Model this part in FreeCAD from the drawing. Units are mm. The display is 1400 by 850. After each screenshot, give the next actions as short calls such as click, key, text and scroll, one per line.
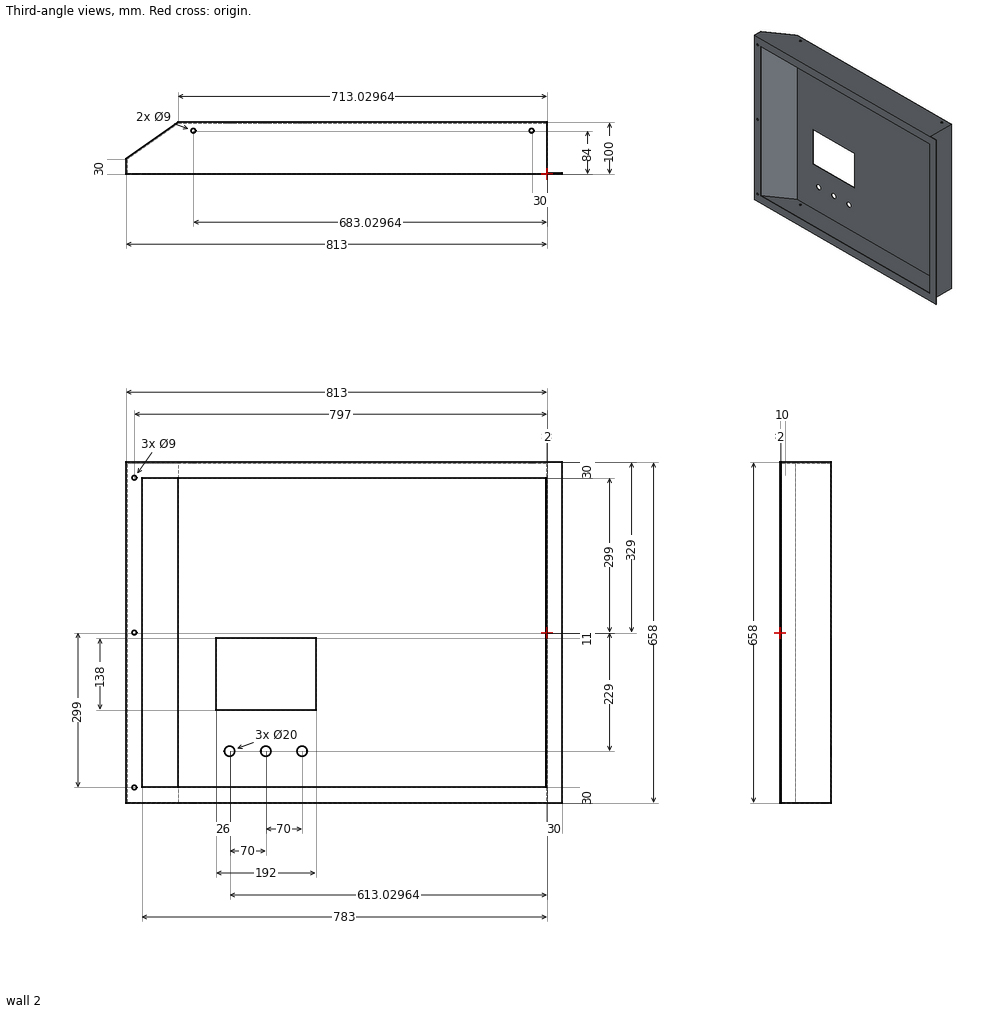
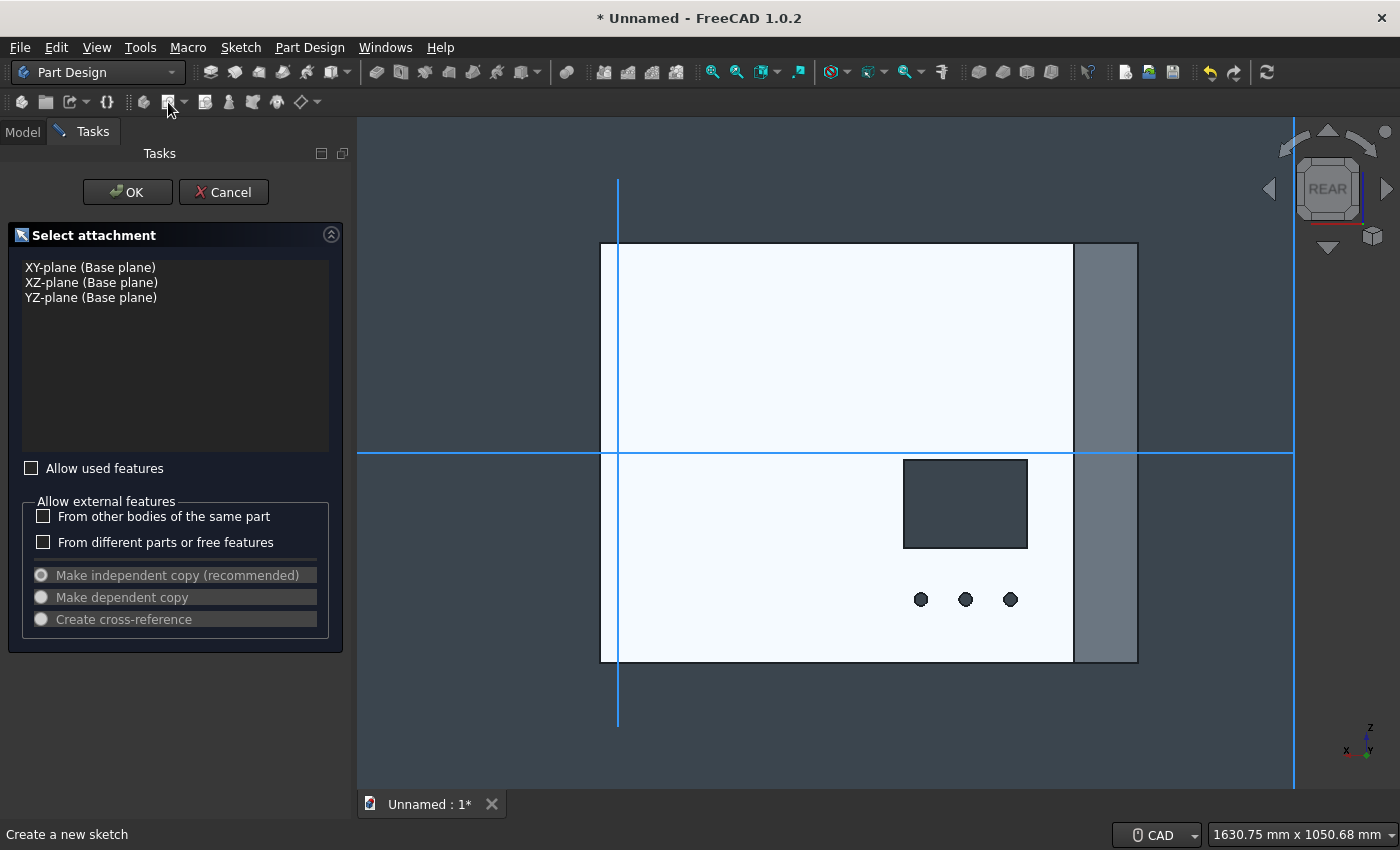
click(82, 282)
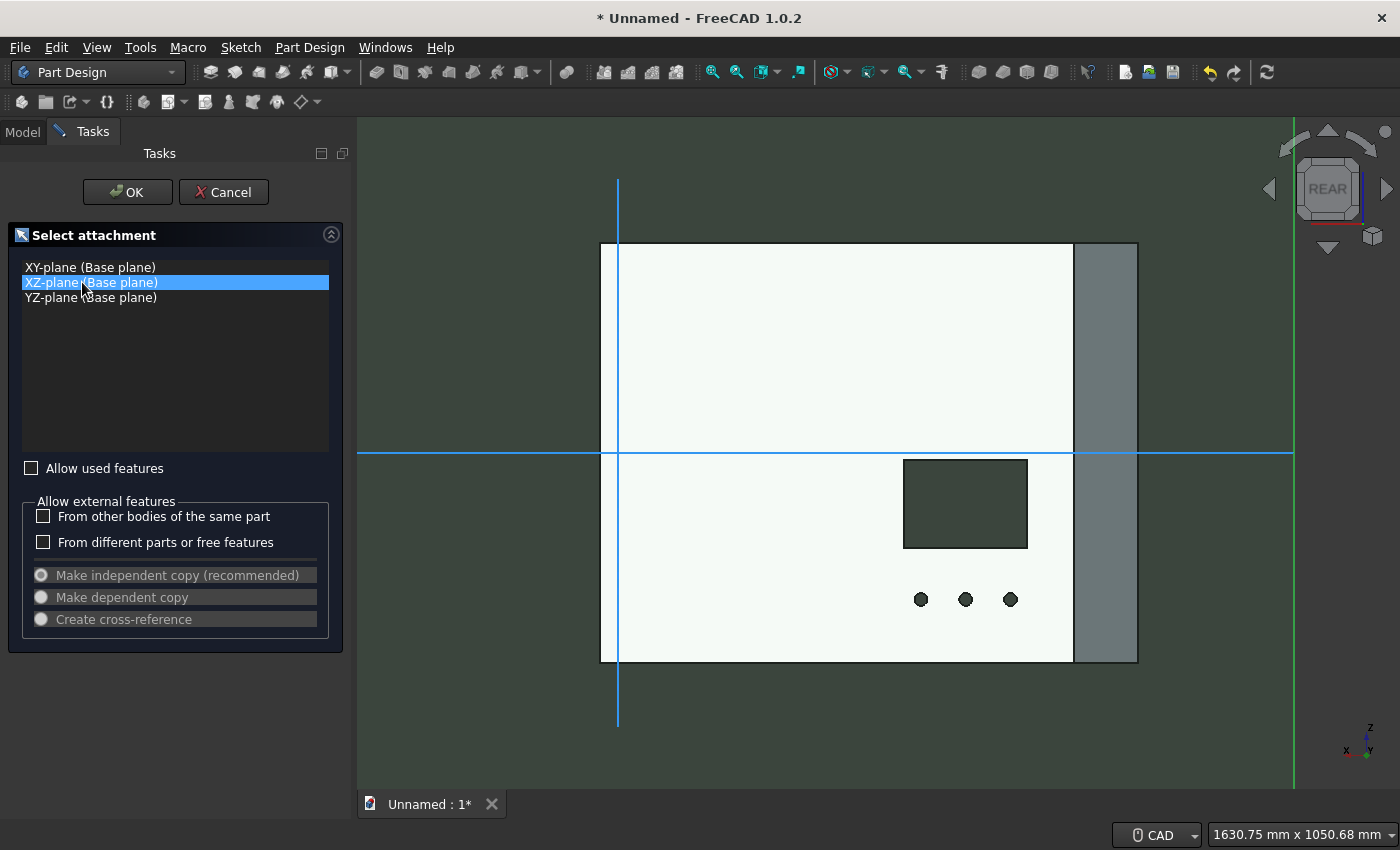
click(128, 192)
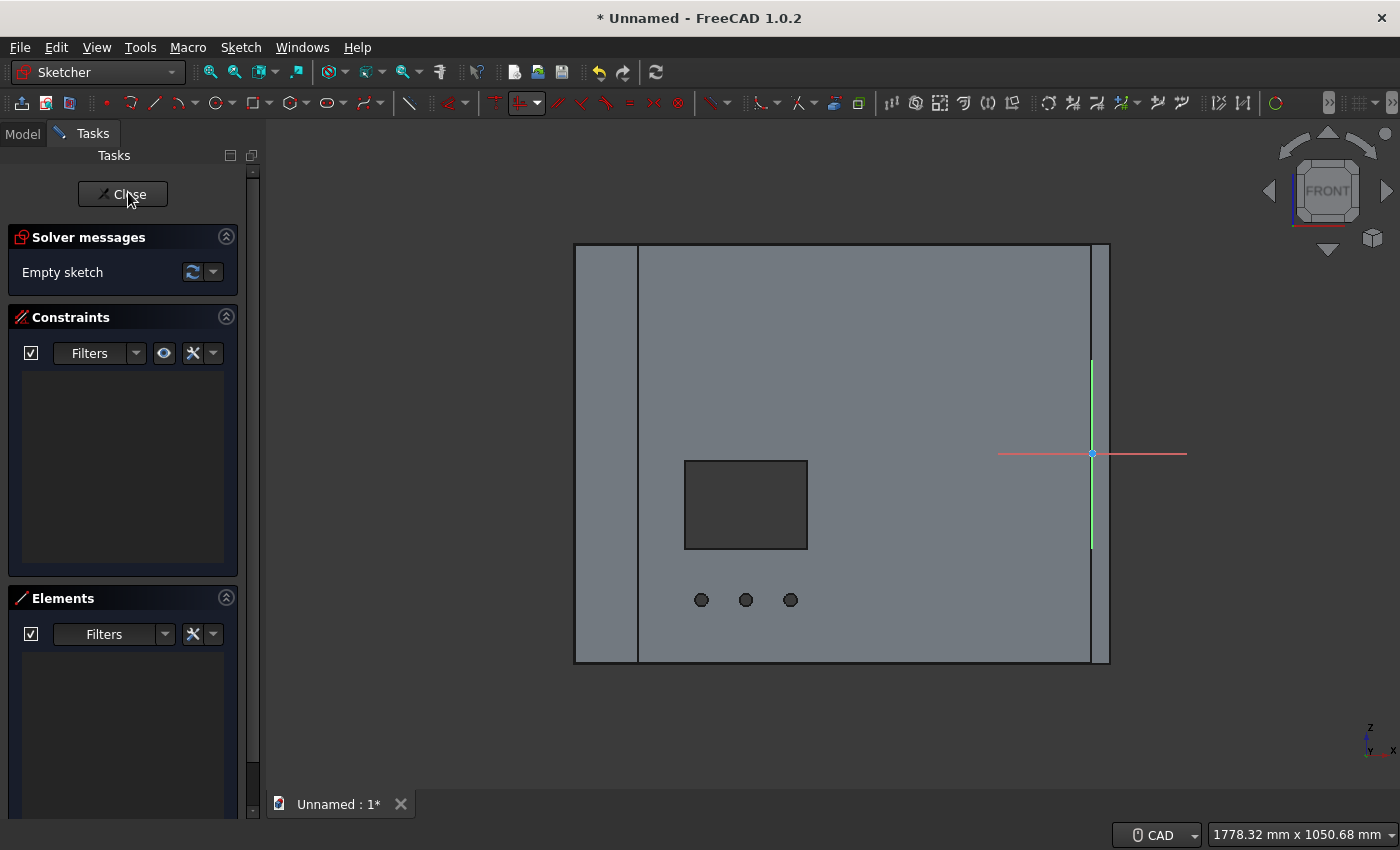
click(132, 104)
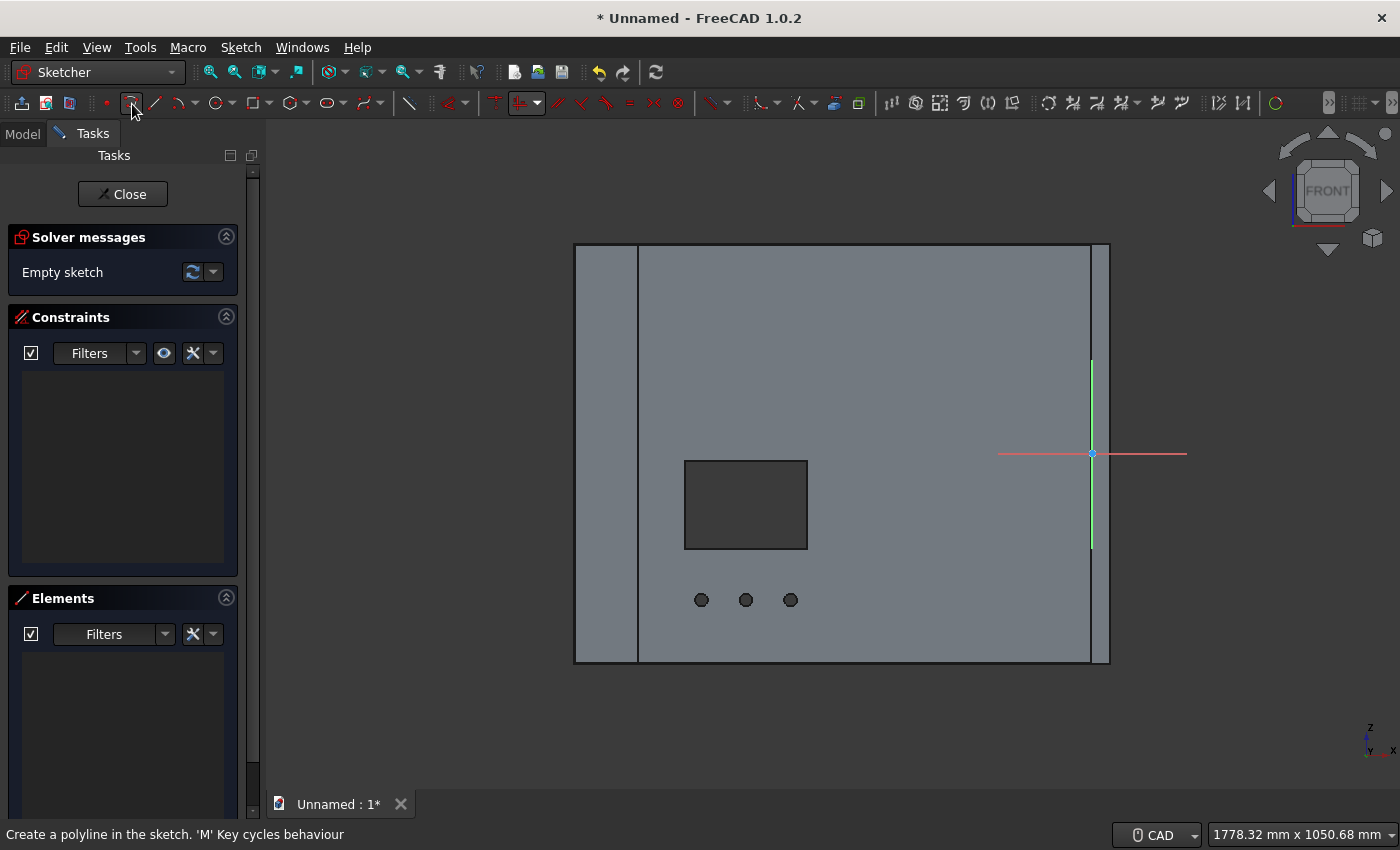
click(1092, 263)
click(1083, 244)
click(574, 244)
click(574, 664)
click(1092, 664)
click(1083, 645)
click(593, 645)
click(593, 263)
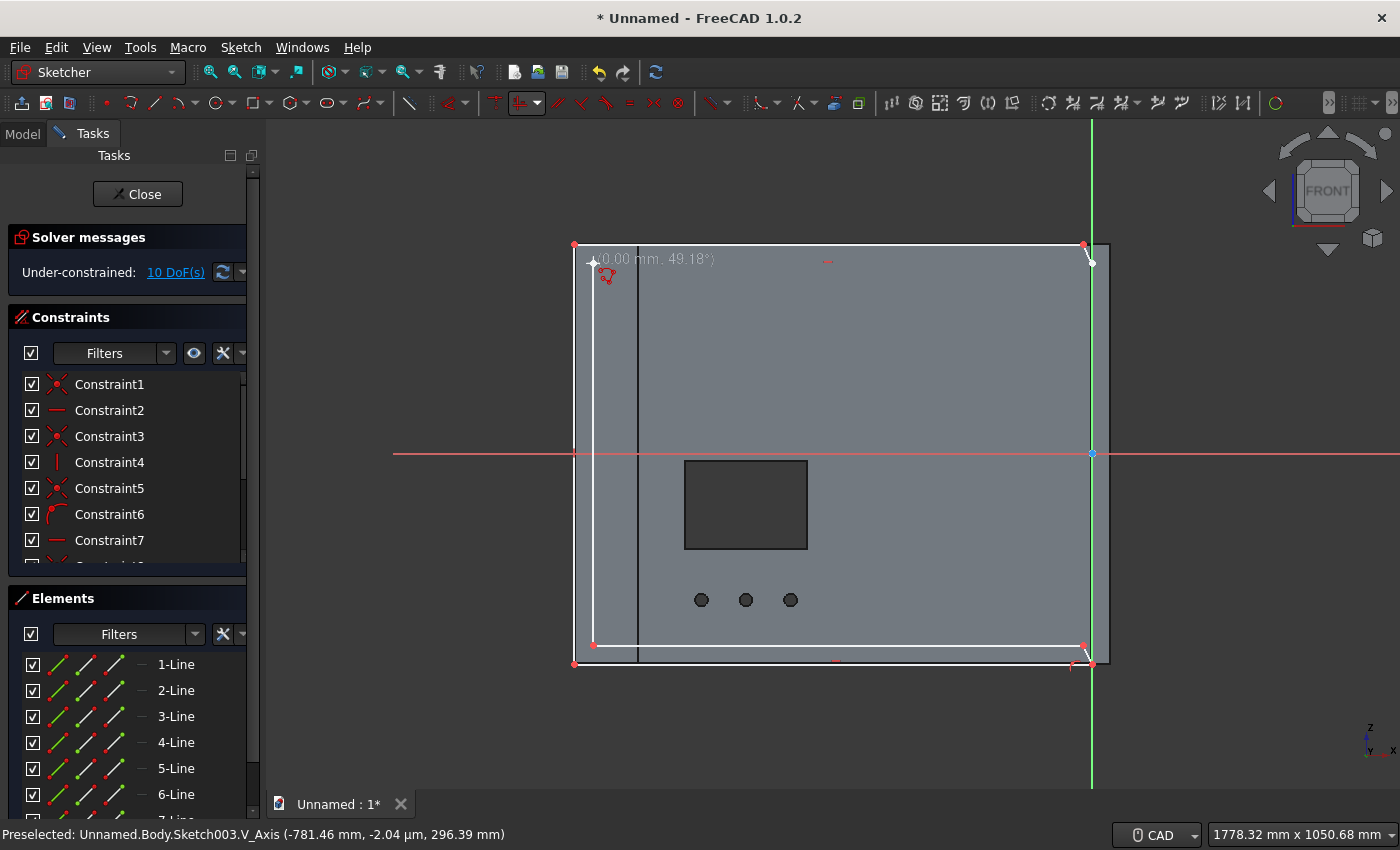
scroll(1092, 263, up, 3)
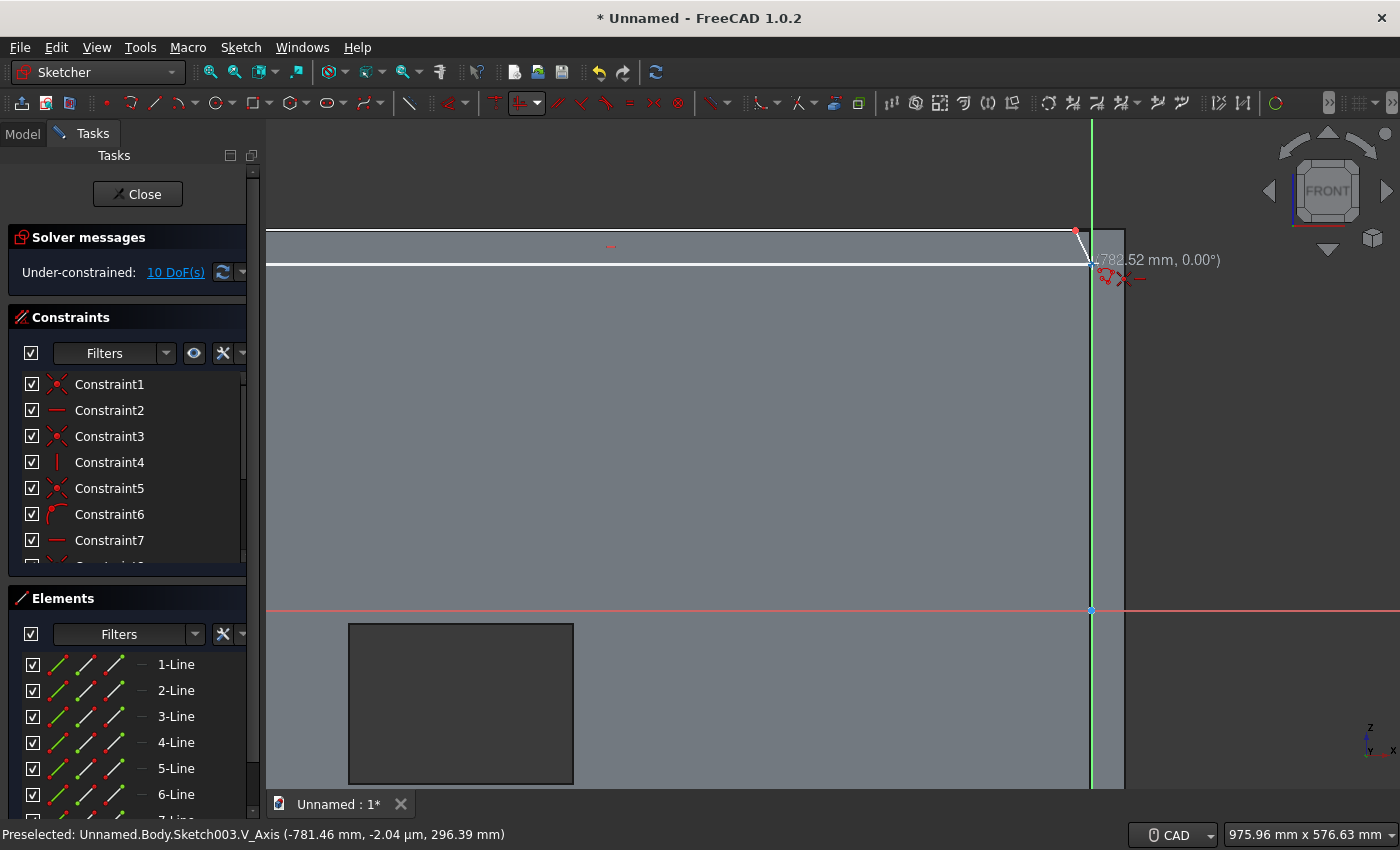
click(1091, 265)
key(Escape)
key(Escape)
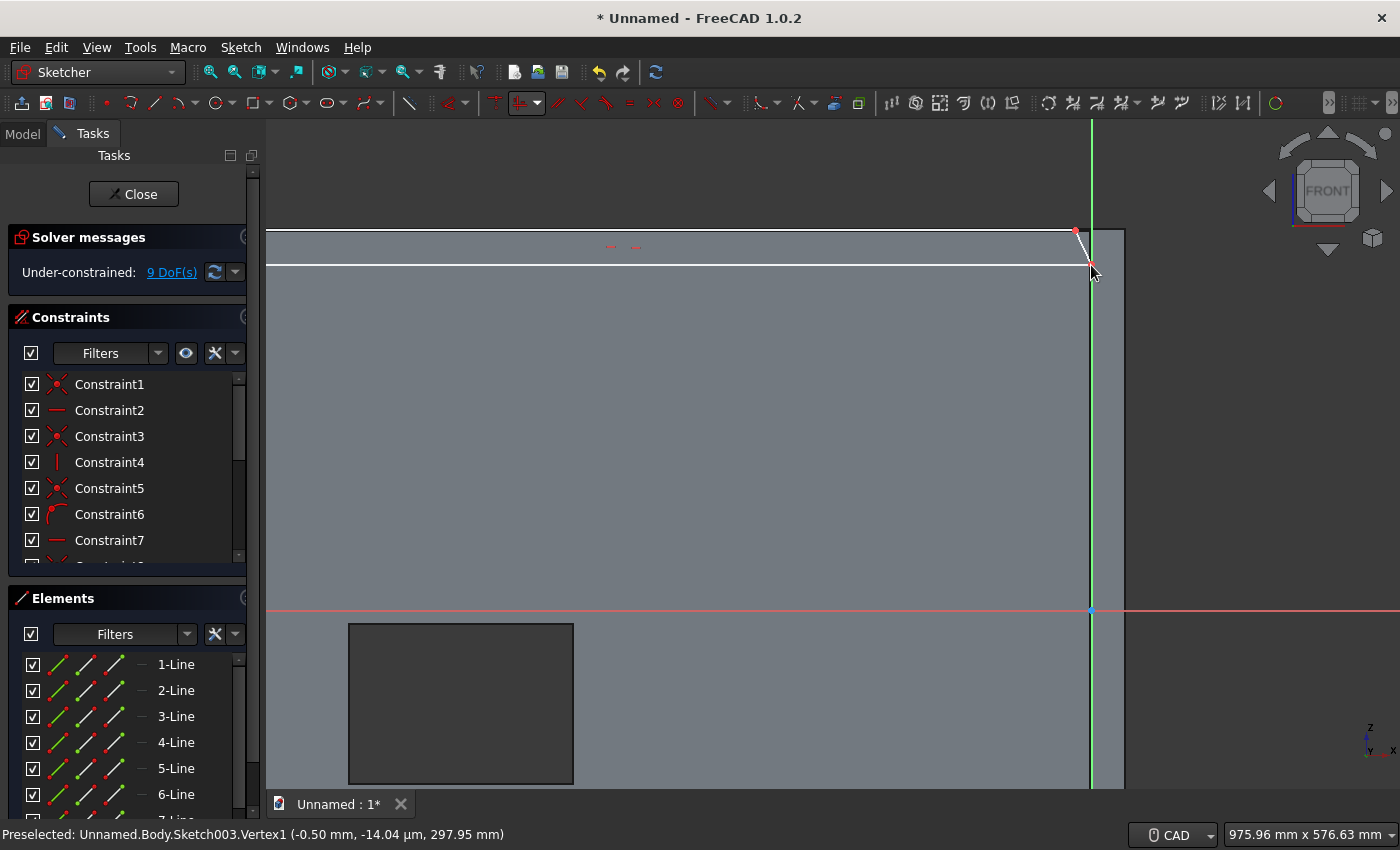
click(1080, 240)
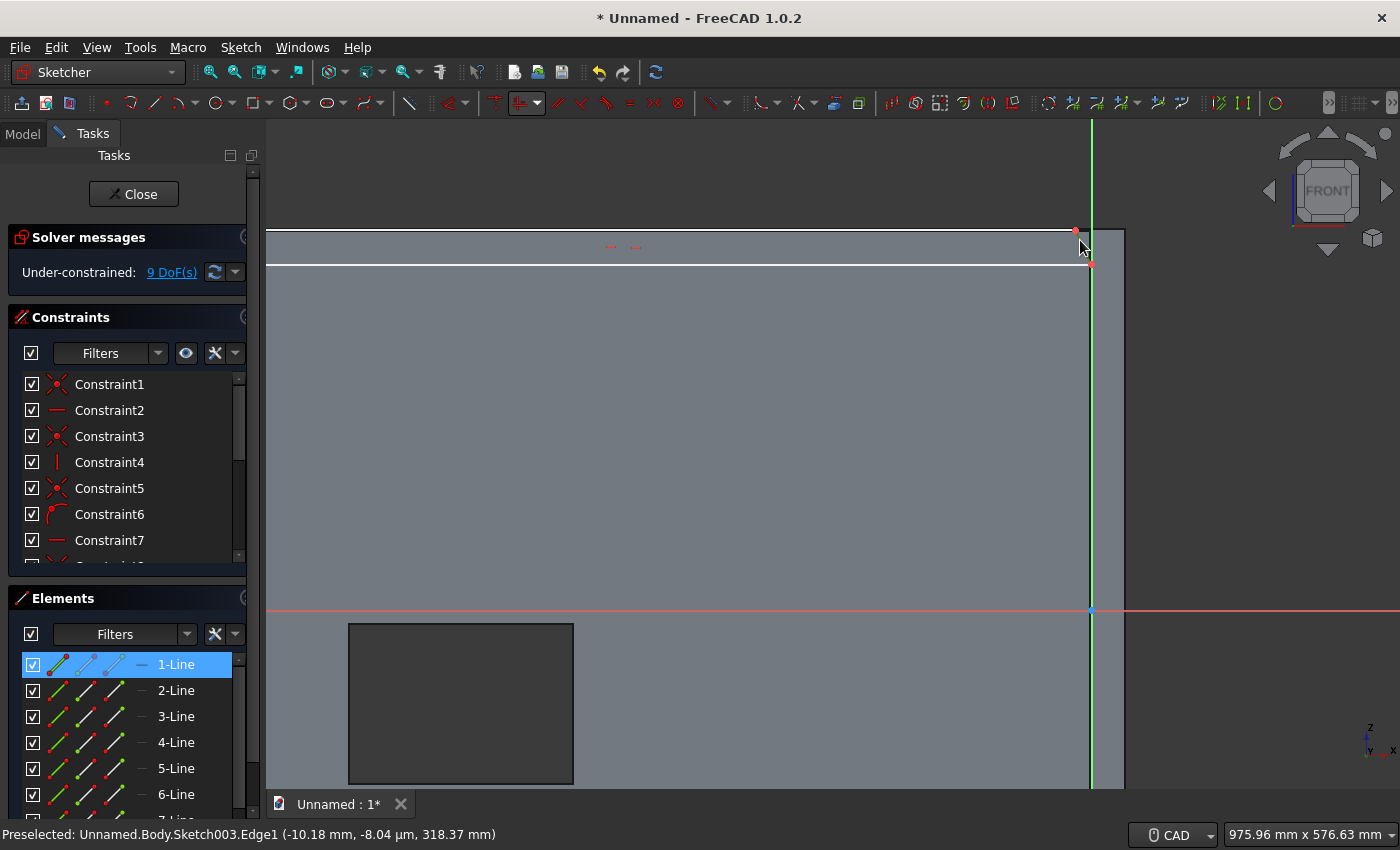
key(v)